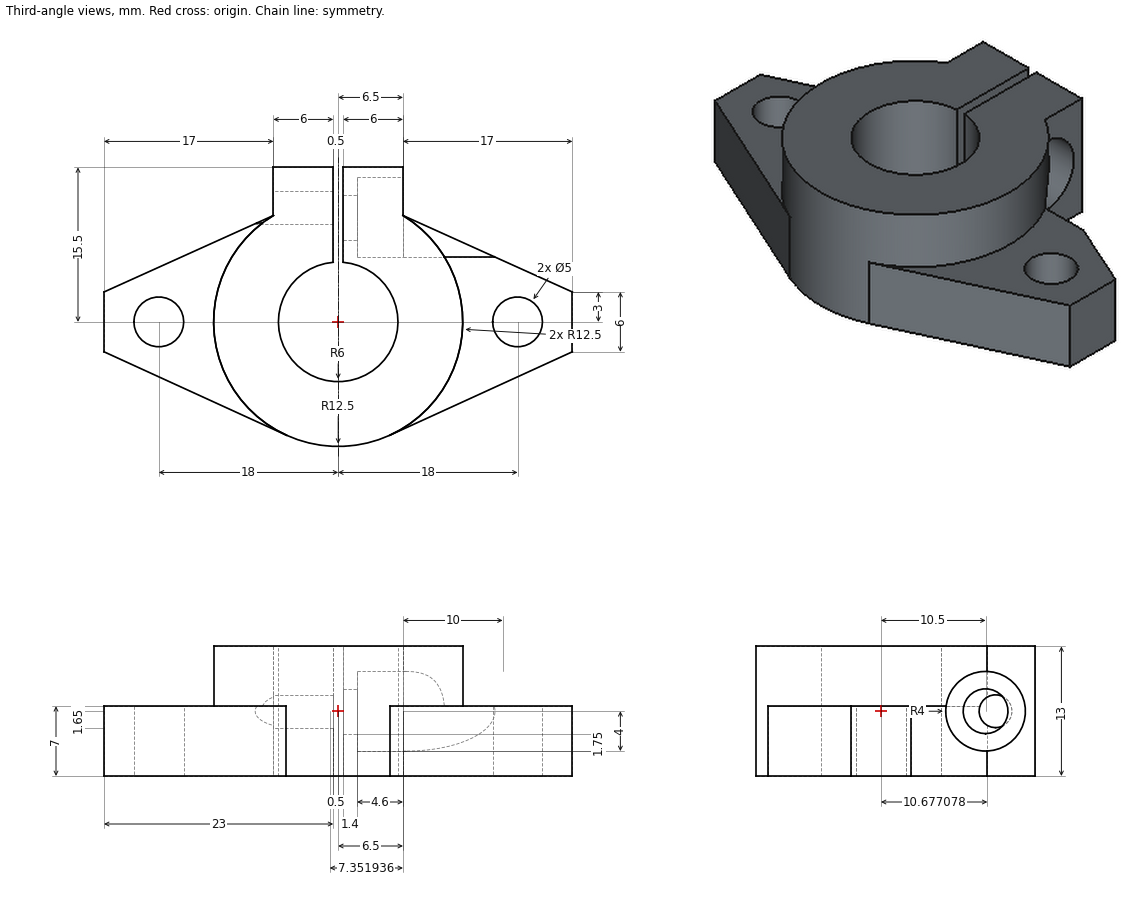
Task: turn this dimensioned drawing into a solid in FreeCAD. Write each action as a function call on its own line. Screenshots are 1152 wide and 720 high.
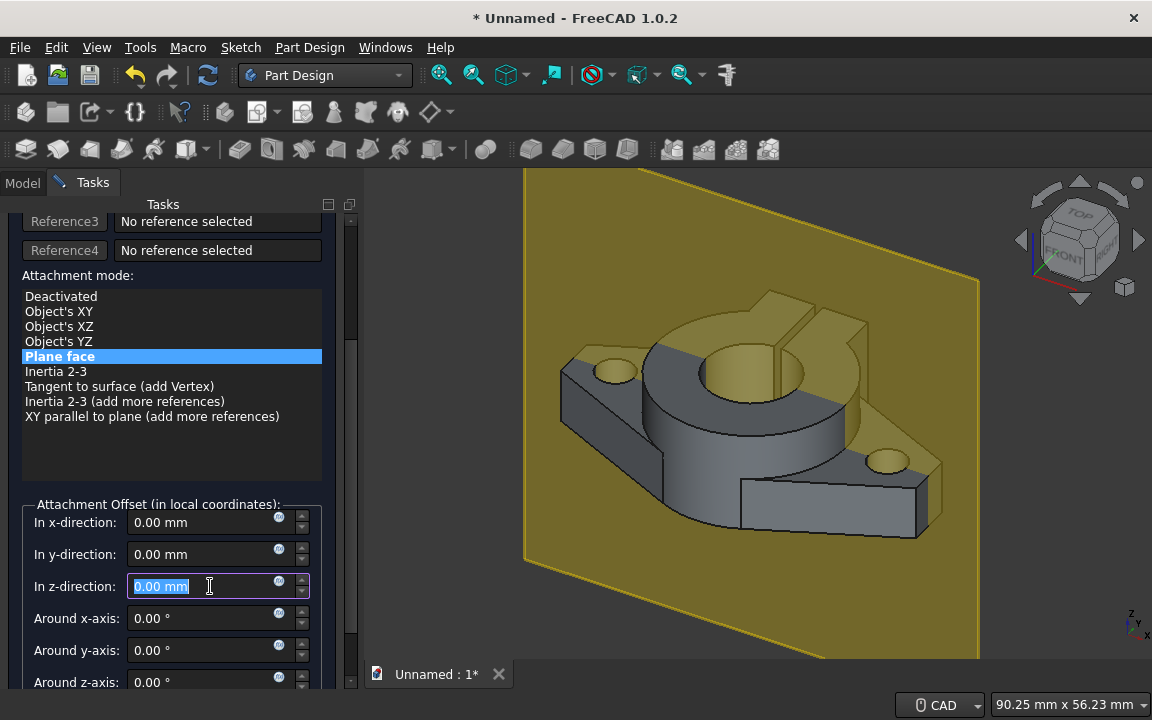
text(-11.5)
key(Tab)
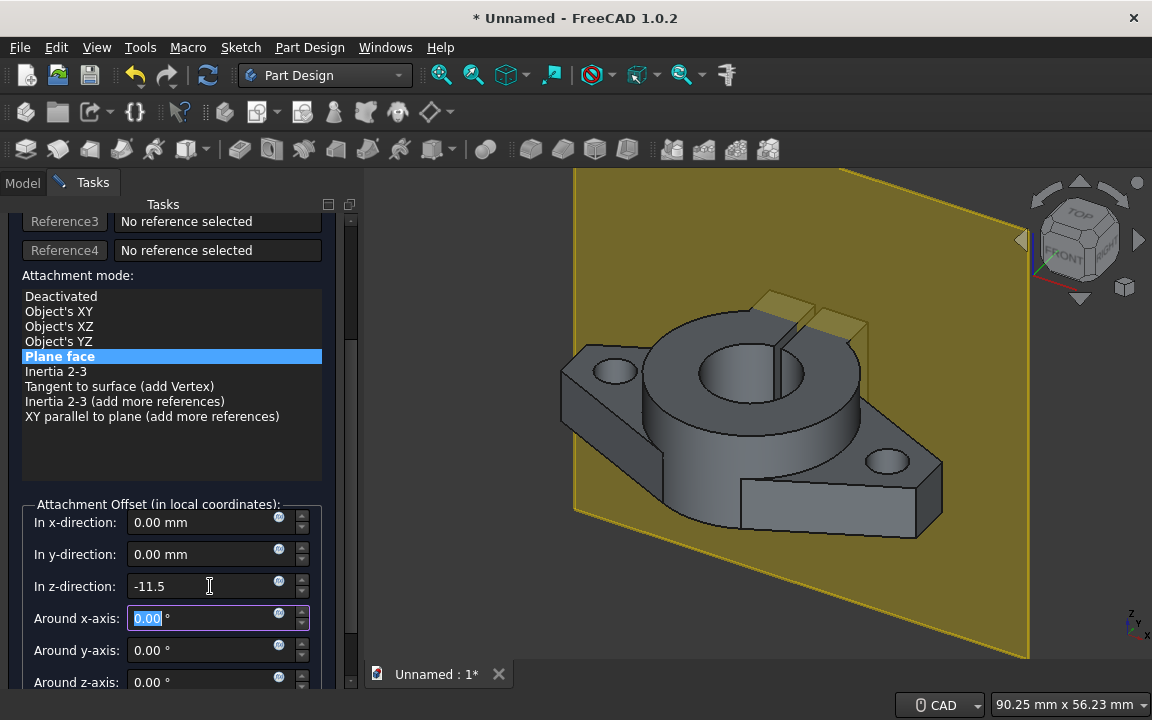
scroll(351, 451, up, 4)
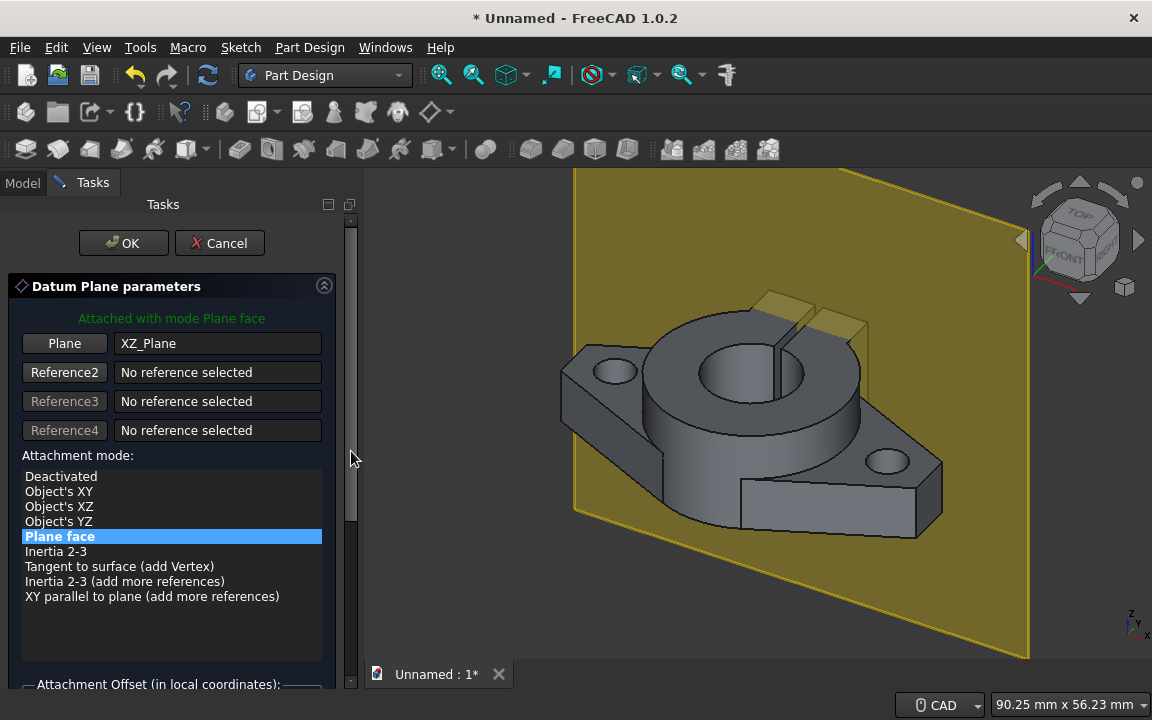
click(124, 243)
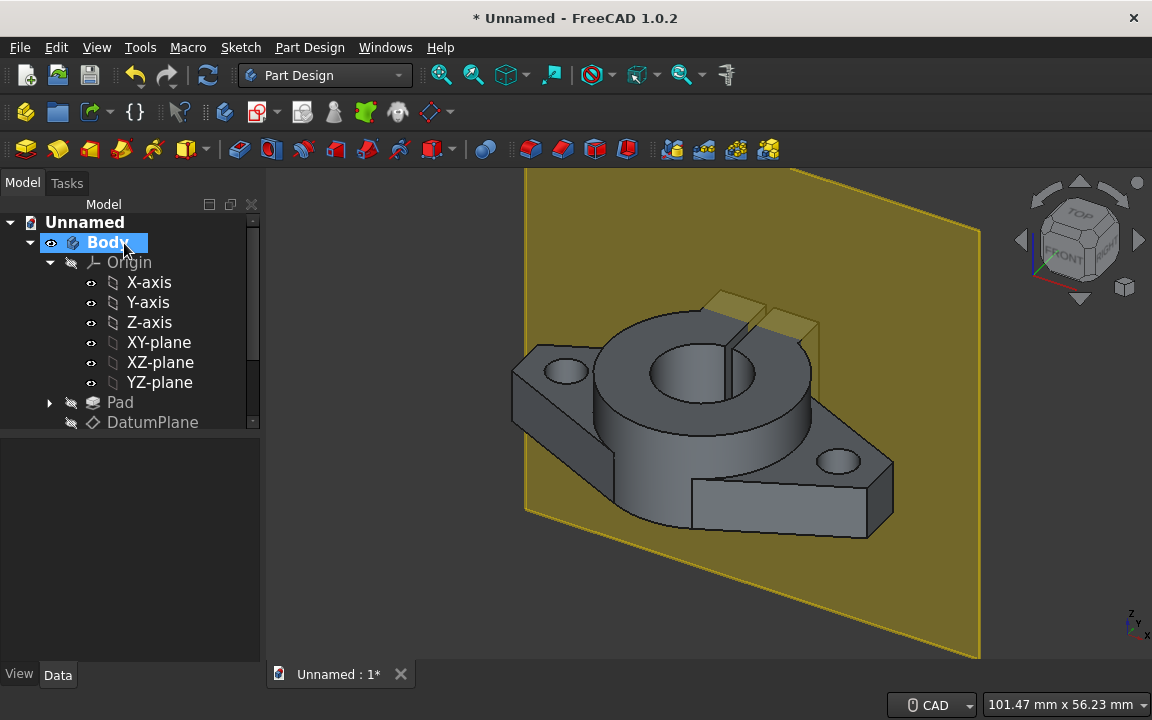
scroll(100, 318, down, 3)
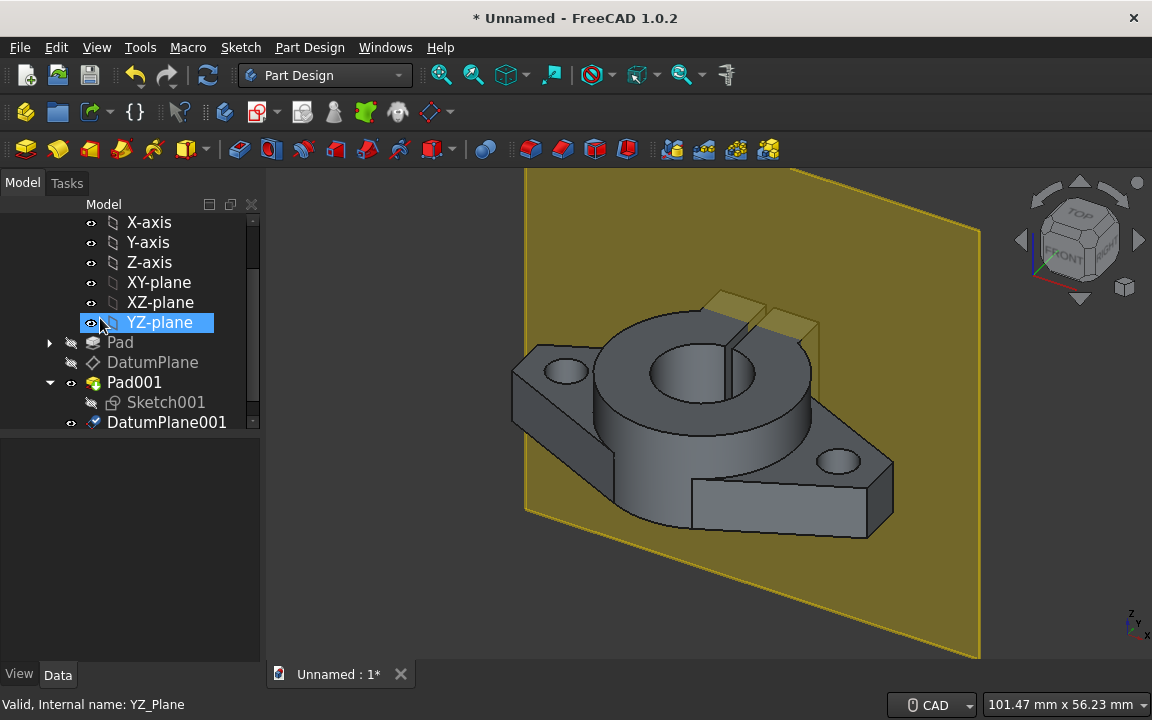
click(116, 403)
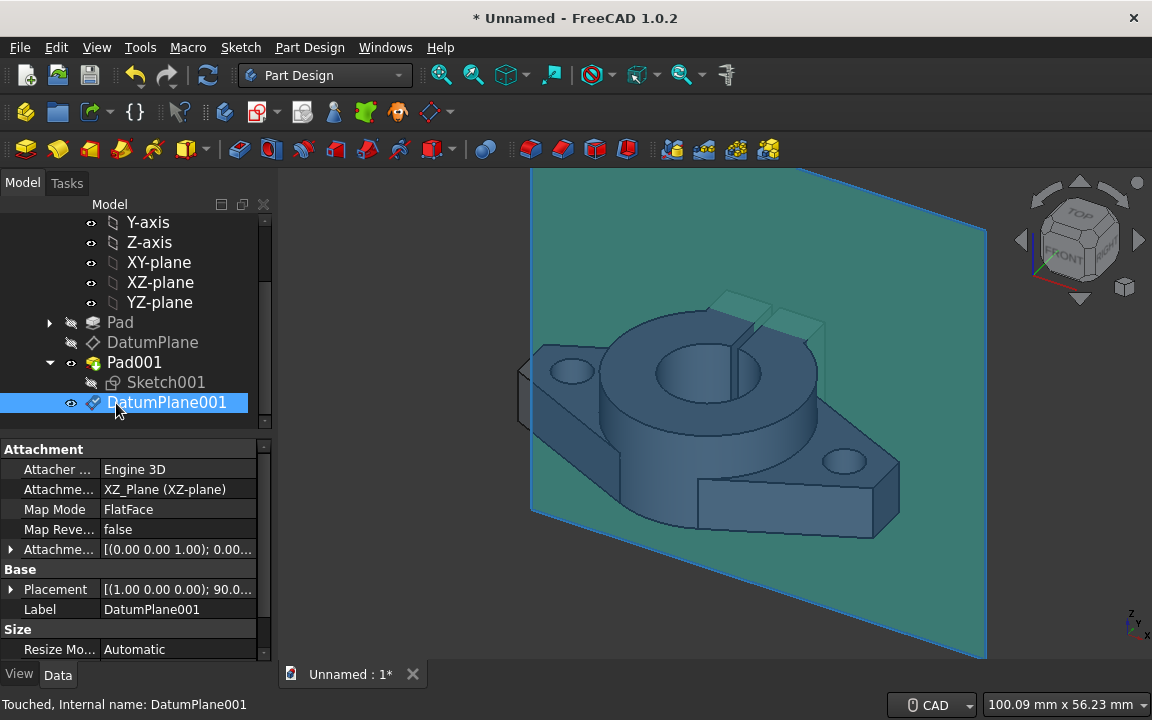
click(258, 112)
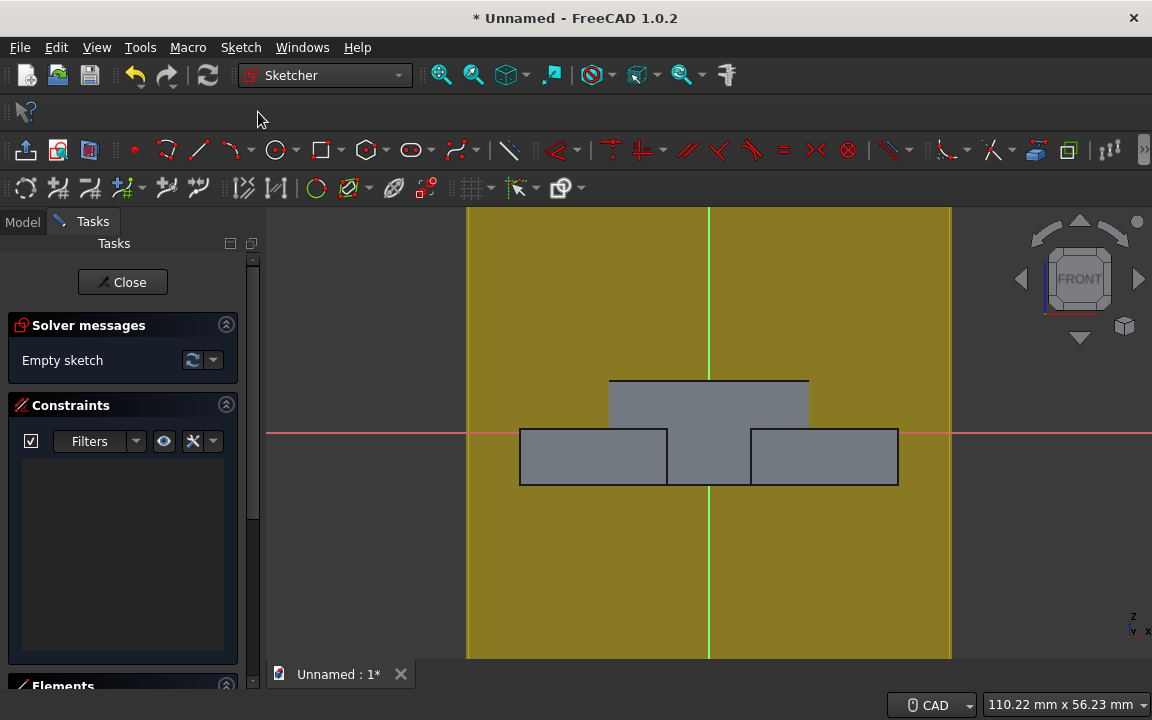
click(90, 150)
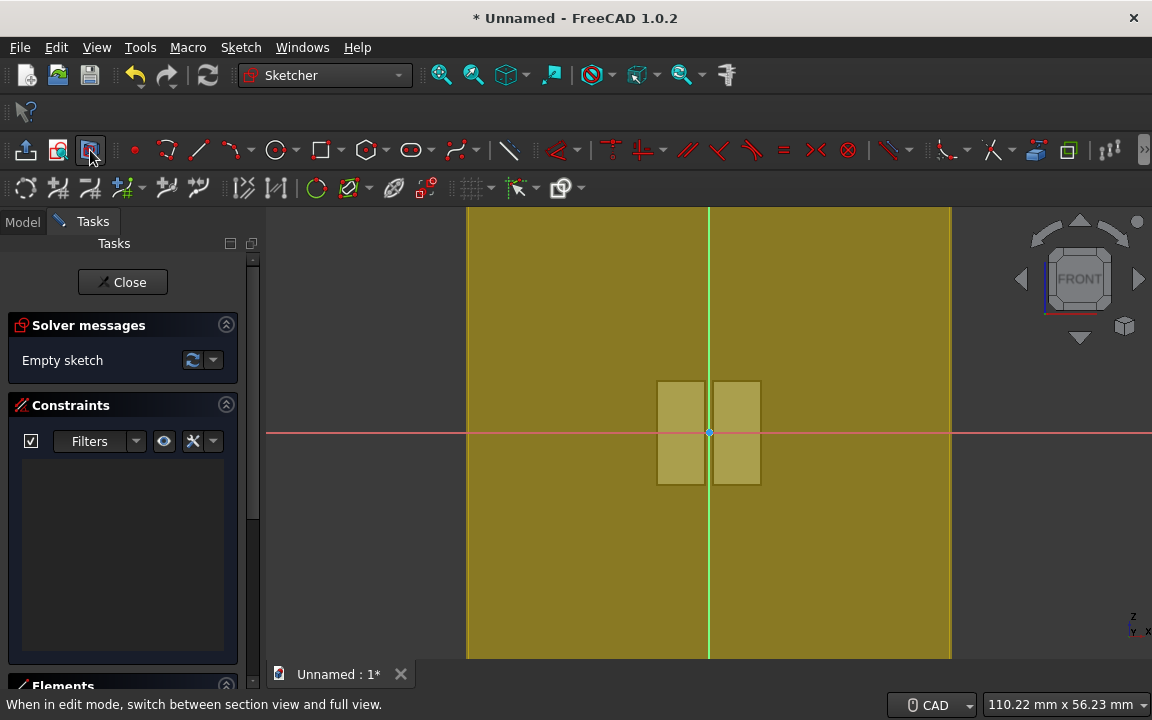
scroll(599, 443, up, 5)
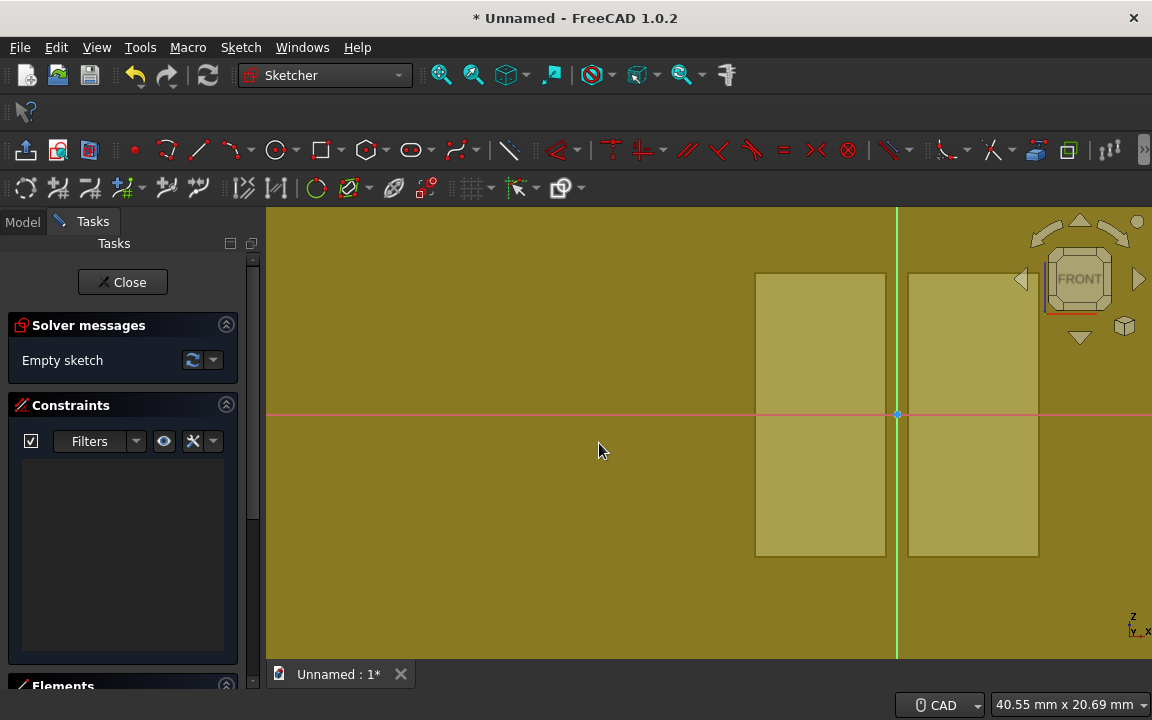
click(322, 150)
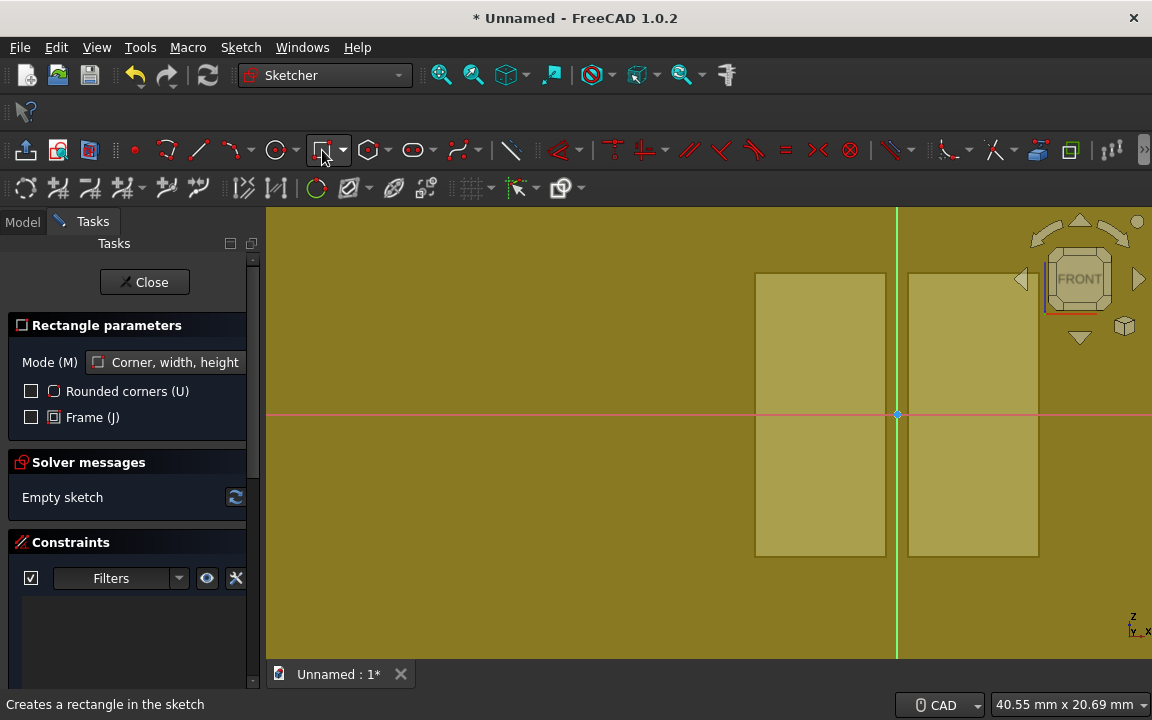
click(384, 415)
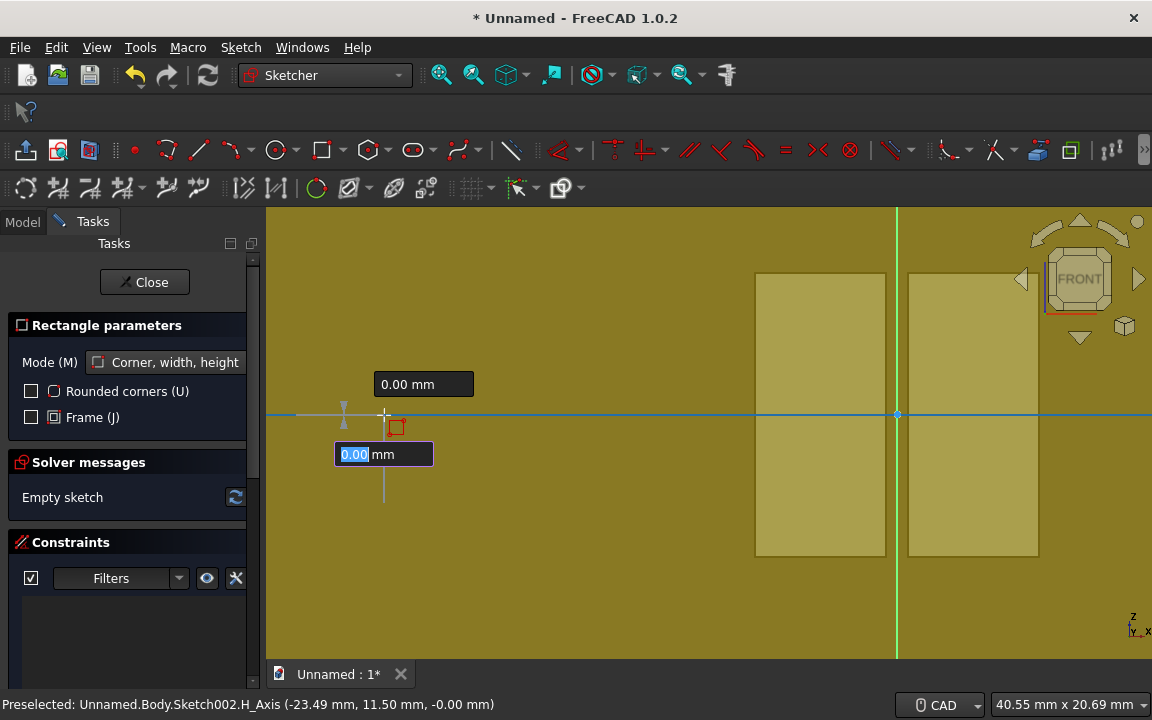
scroll(886, 451, up, 2)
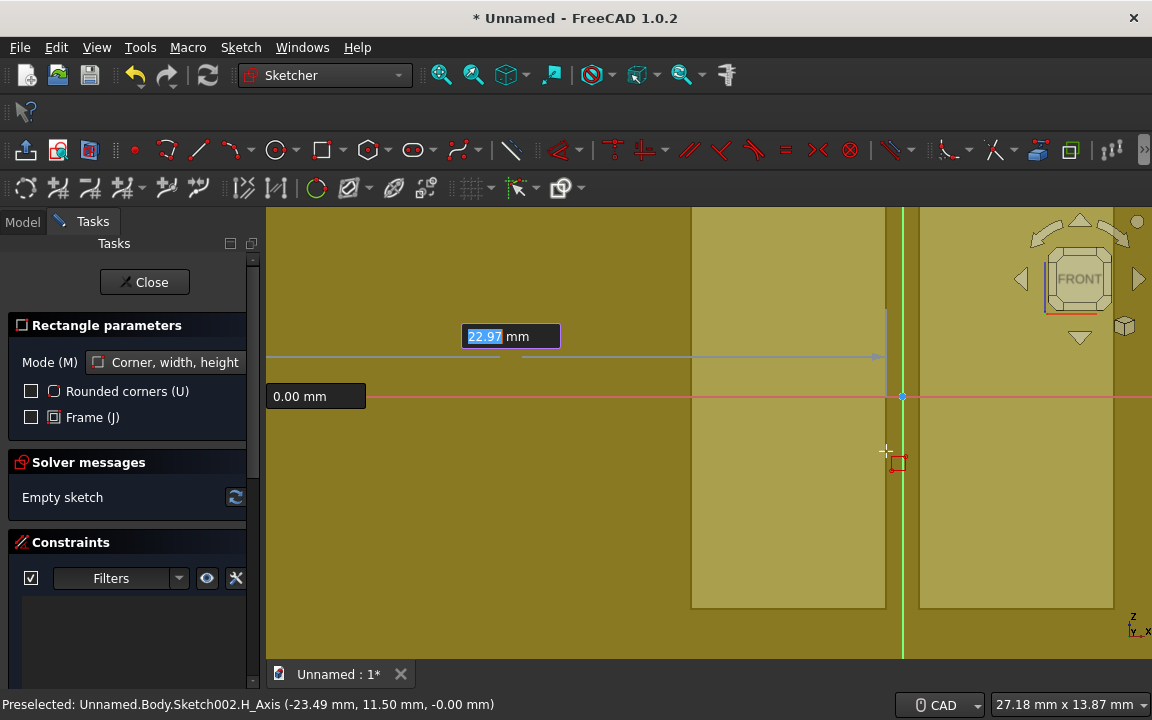
click(886, 451)
key(Escape)